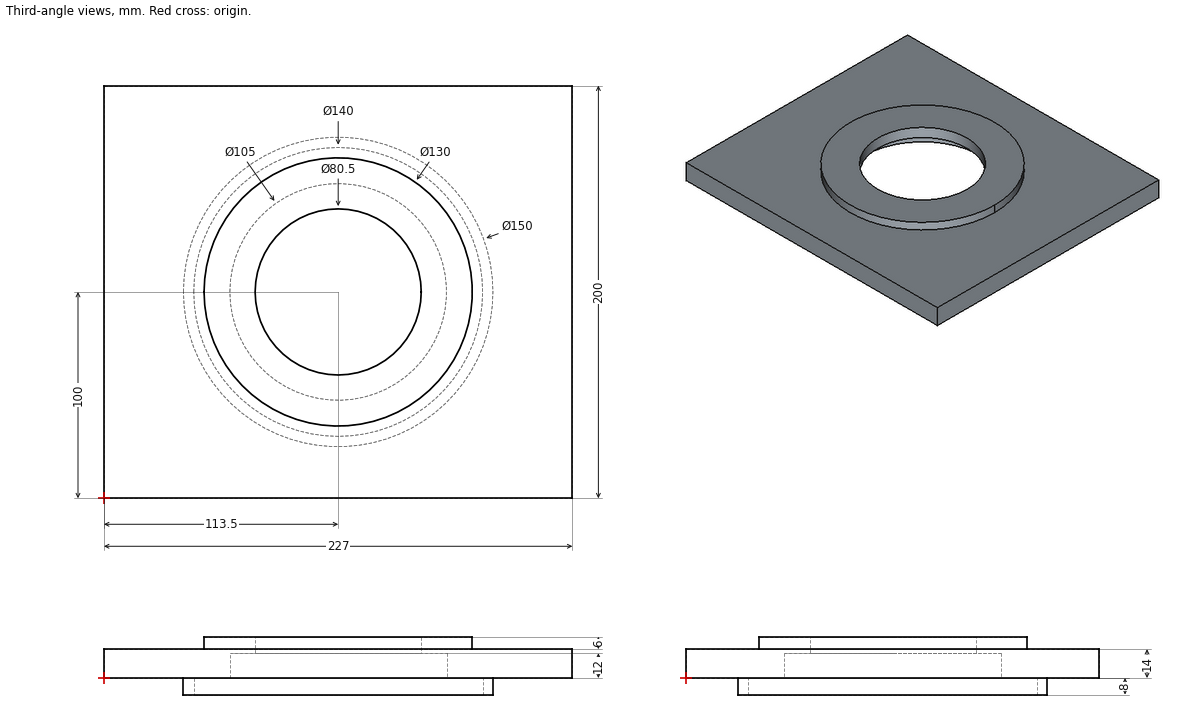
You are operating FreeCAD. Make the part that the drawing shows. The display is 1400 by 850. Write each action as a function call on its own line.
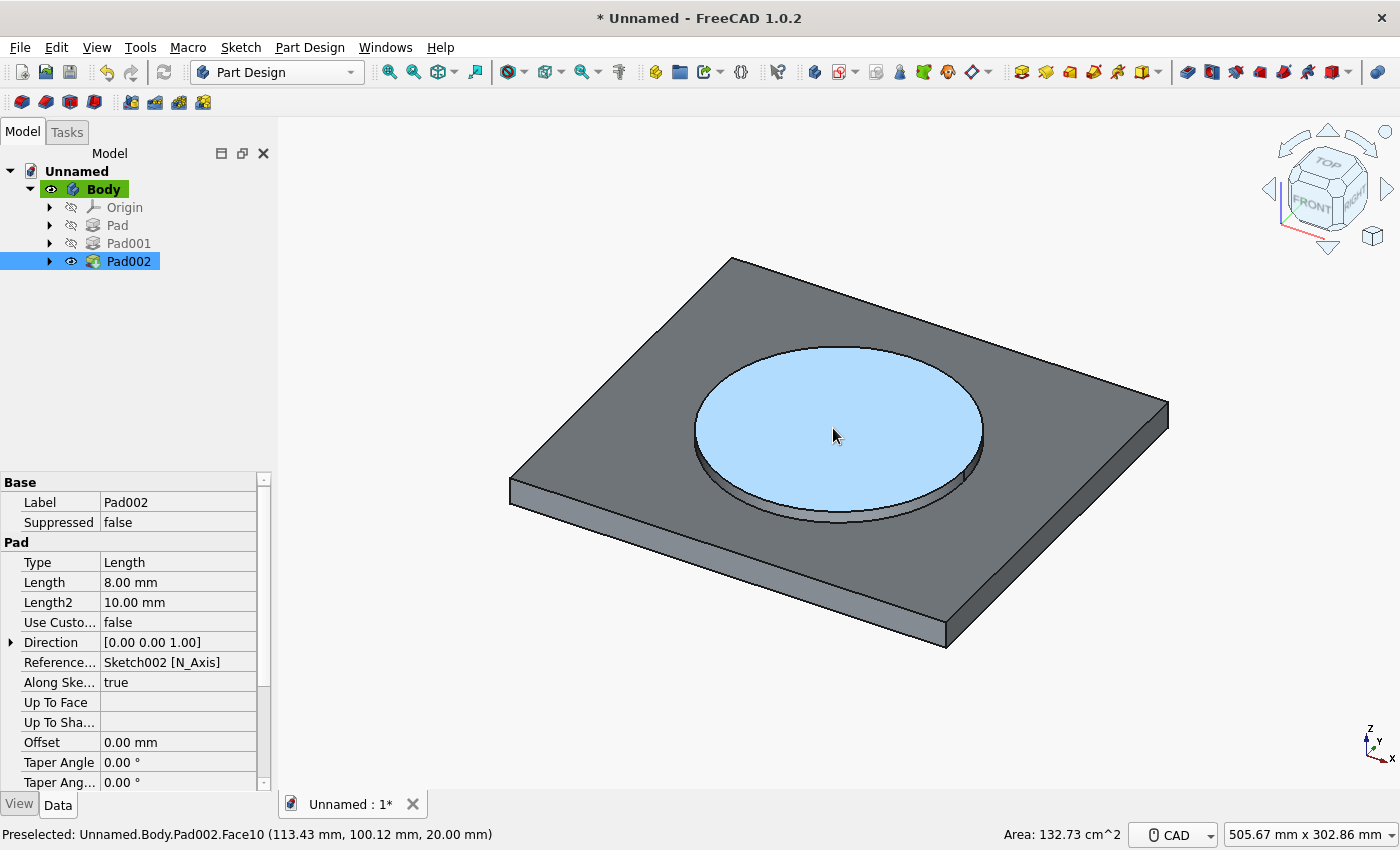
click(840, 72)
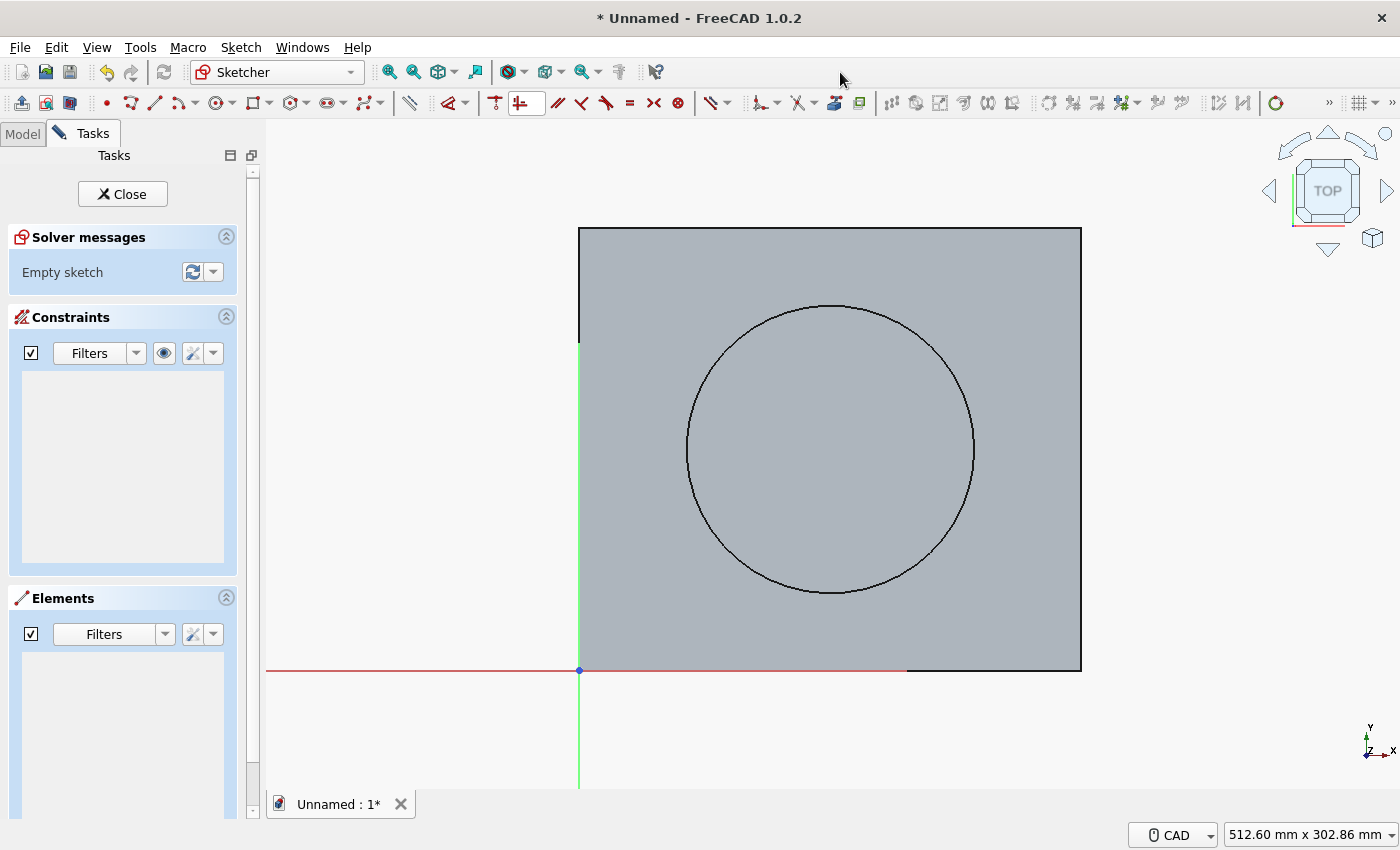
scroll(719, 641, up, 2)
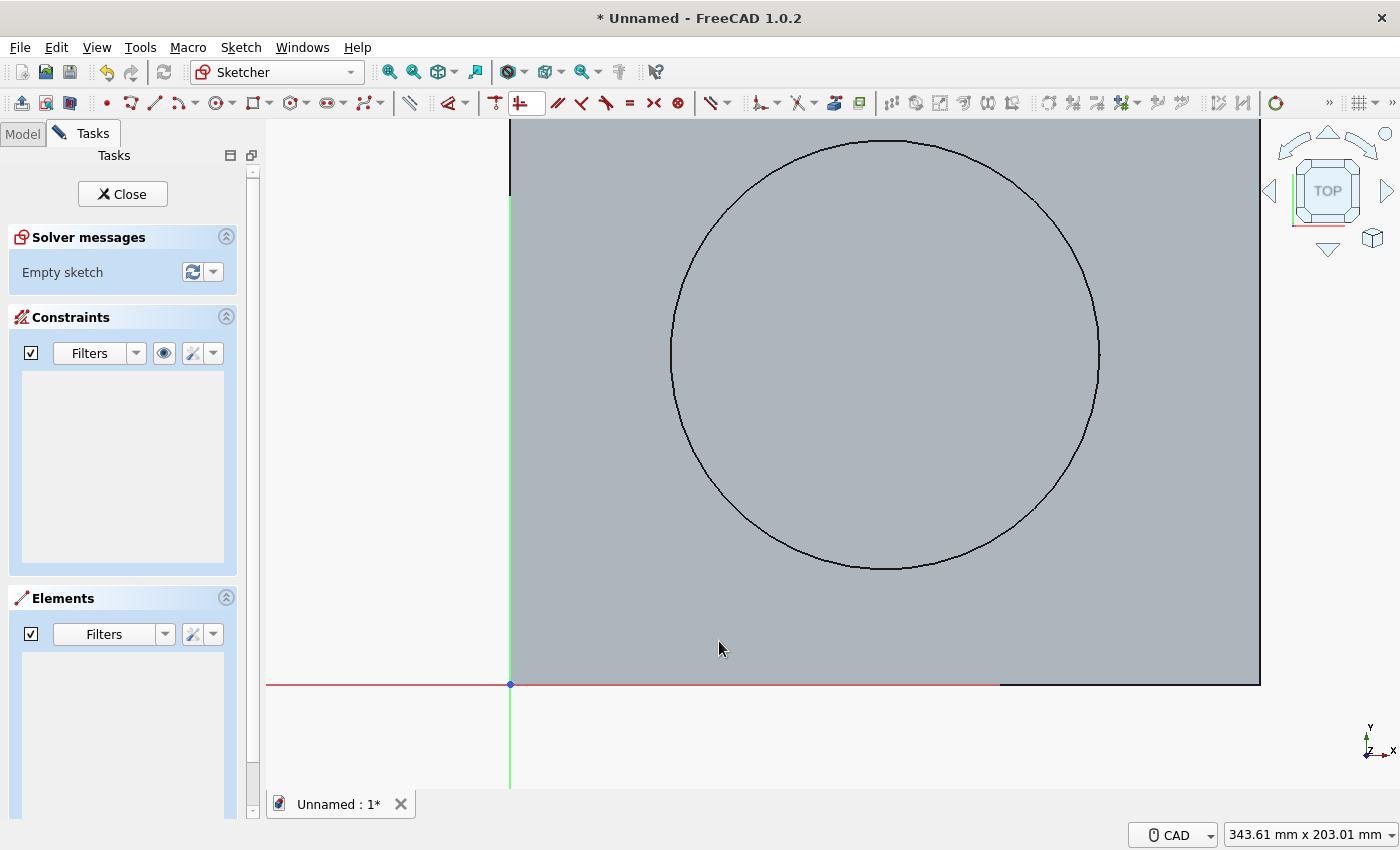
key(g)
key(c)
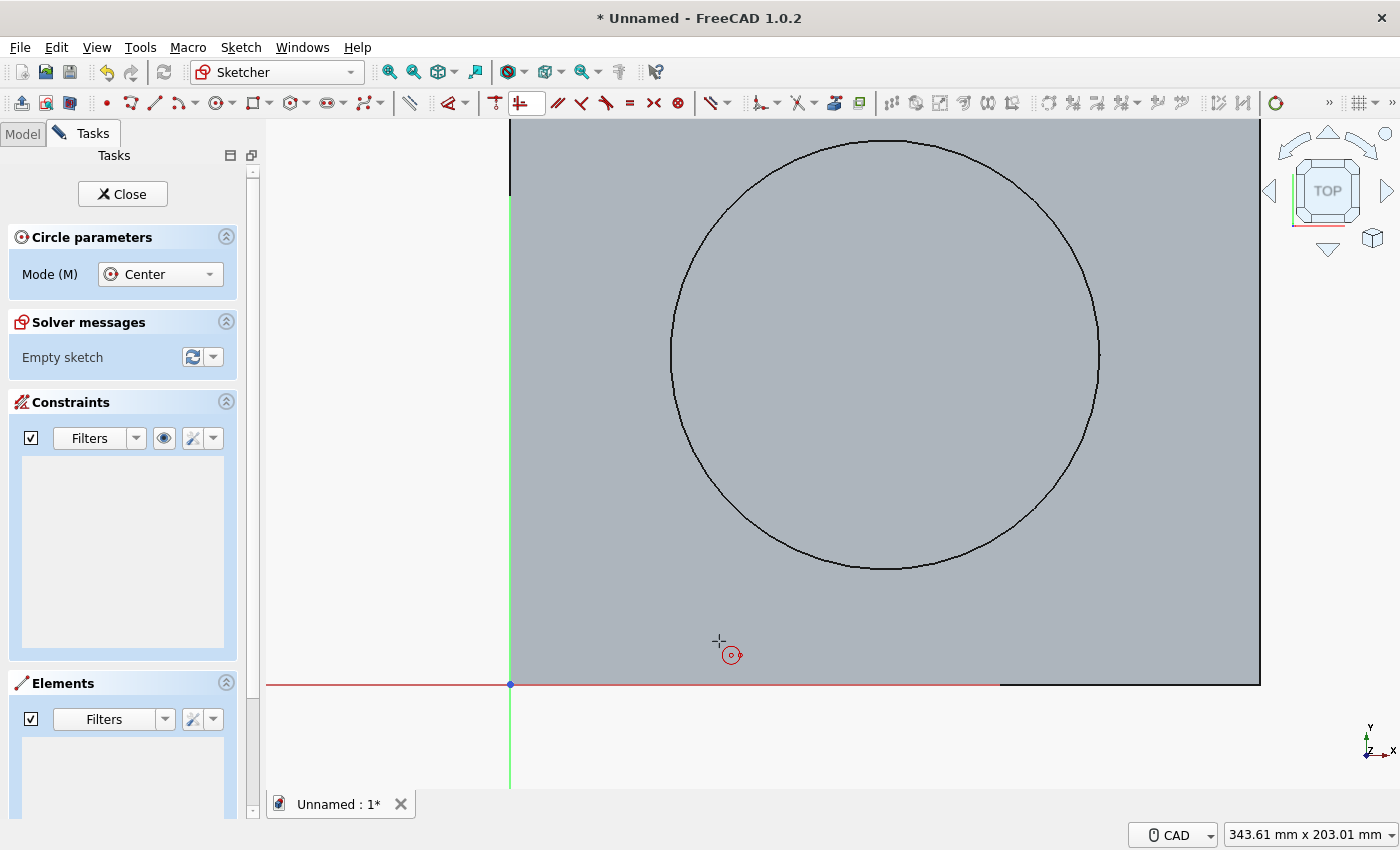
click(885, 355)
click(979, 261)
key(Escape)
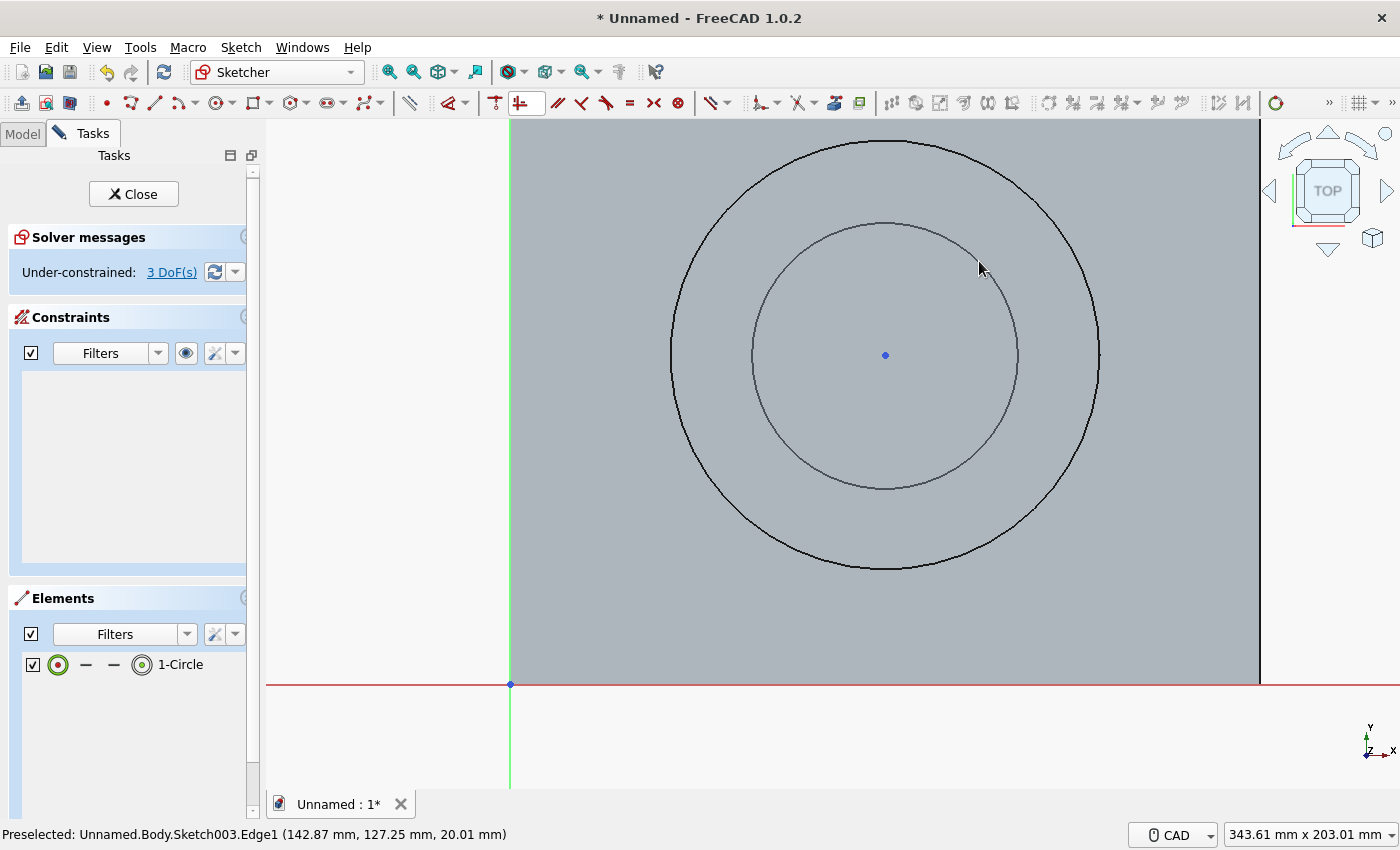
key(d)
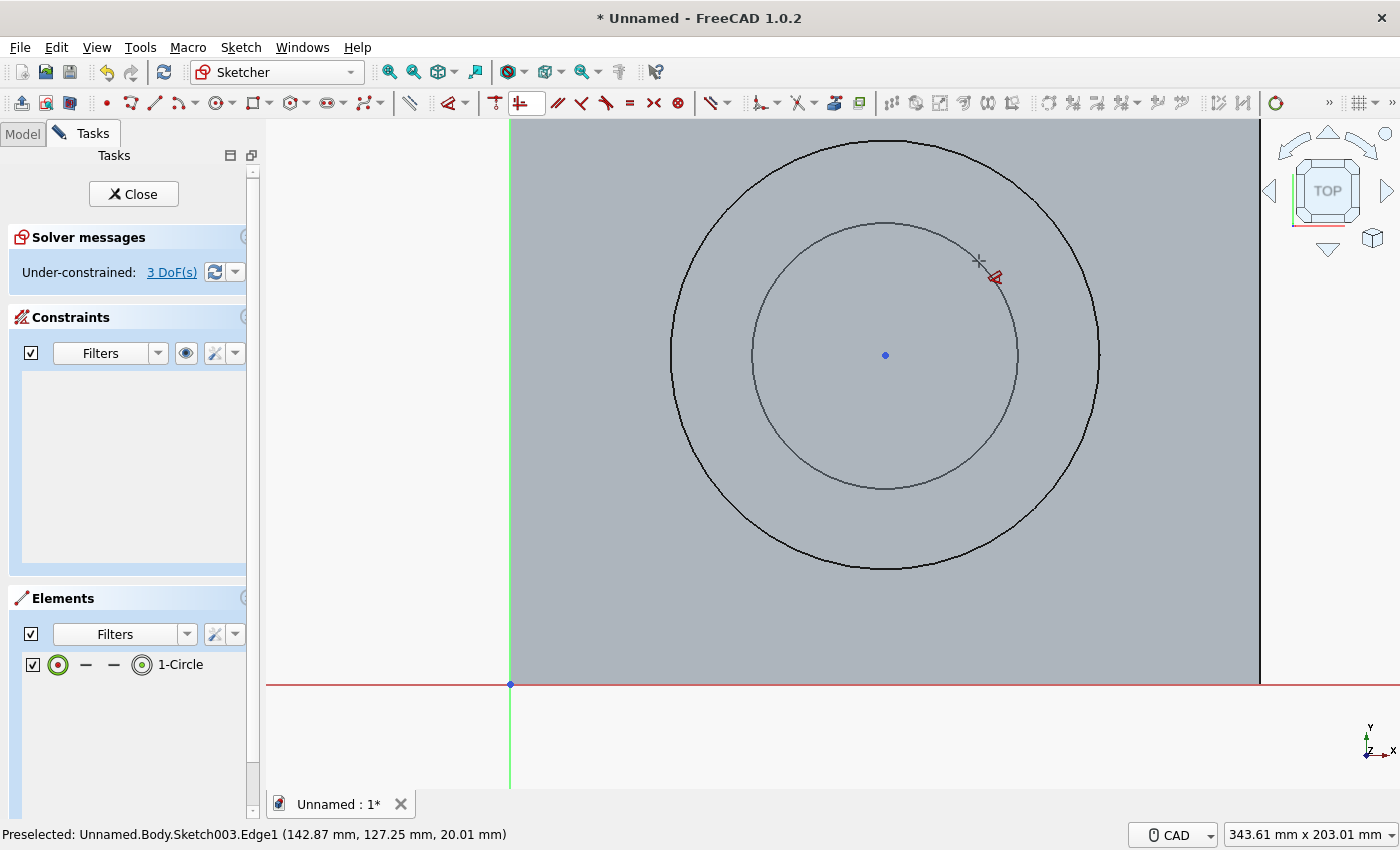
click(979, 262)
click(1002, 239)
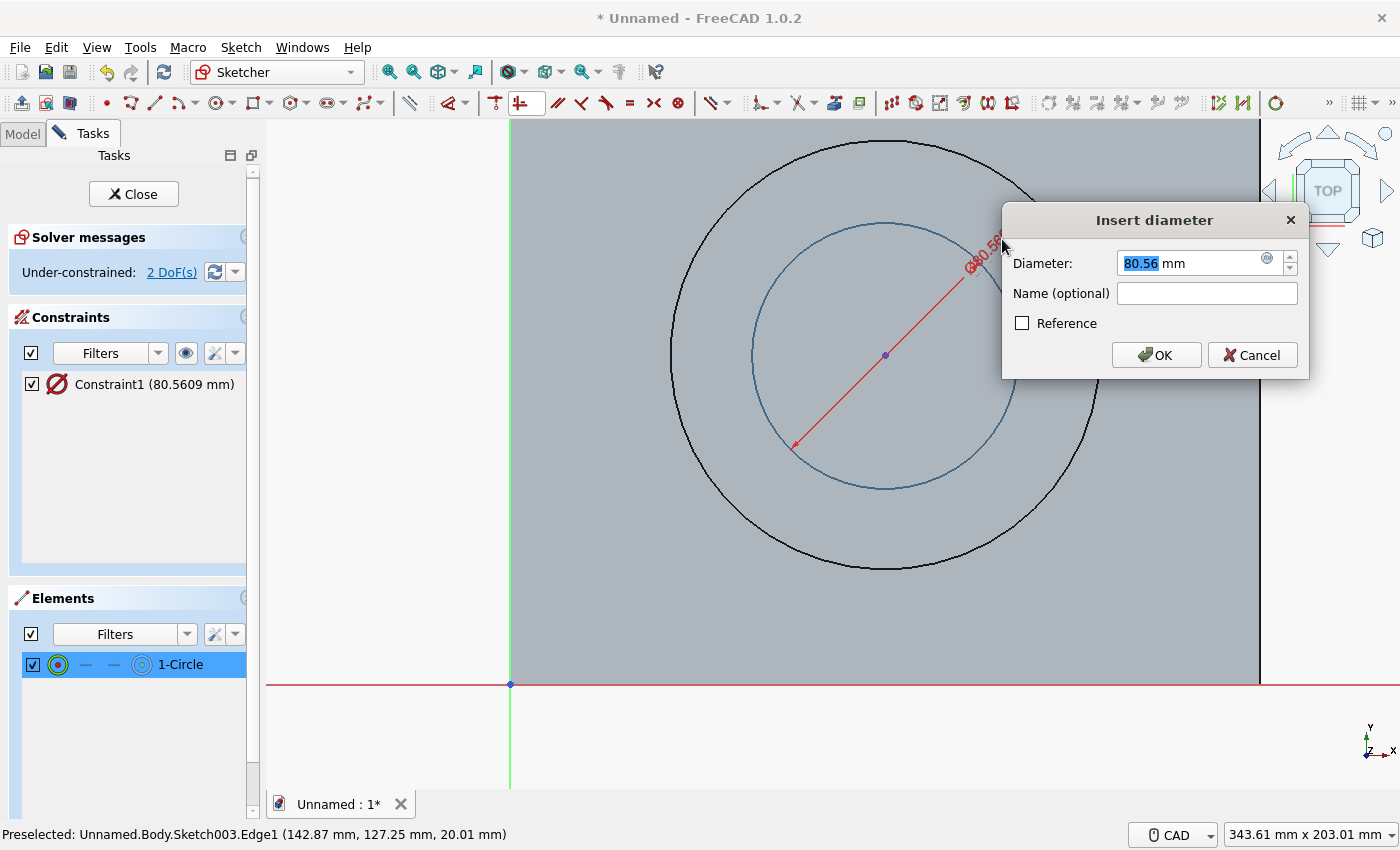
text(80.5)
key(Return)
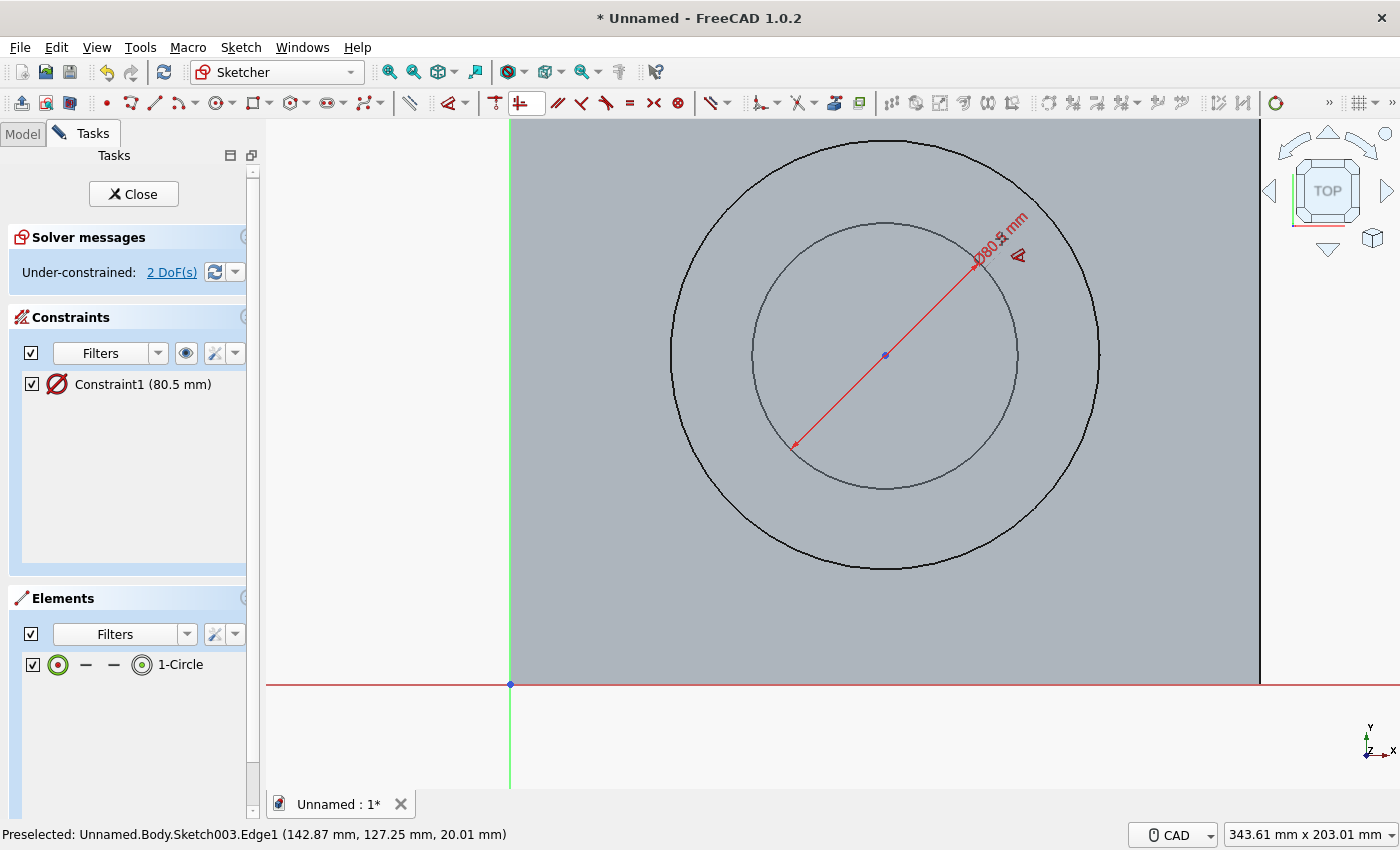
click(885, 356)
click(476, 520)